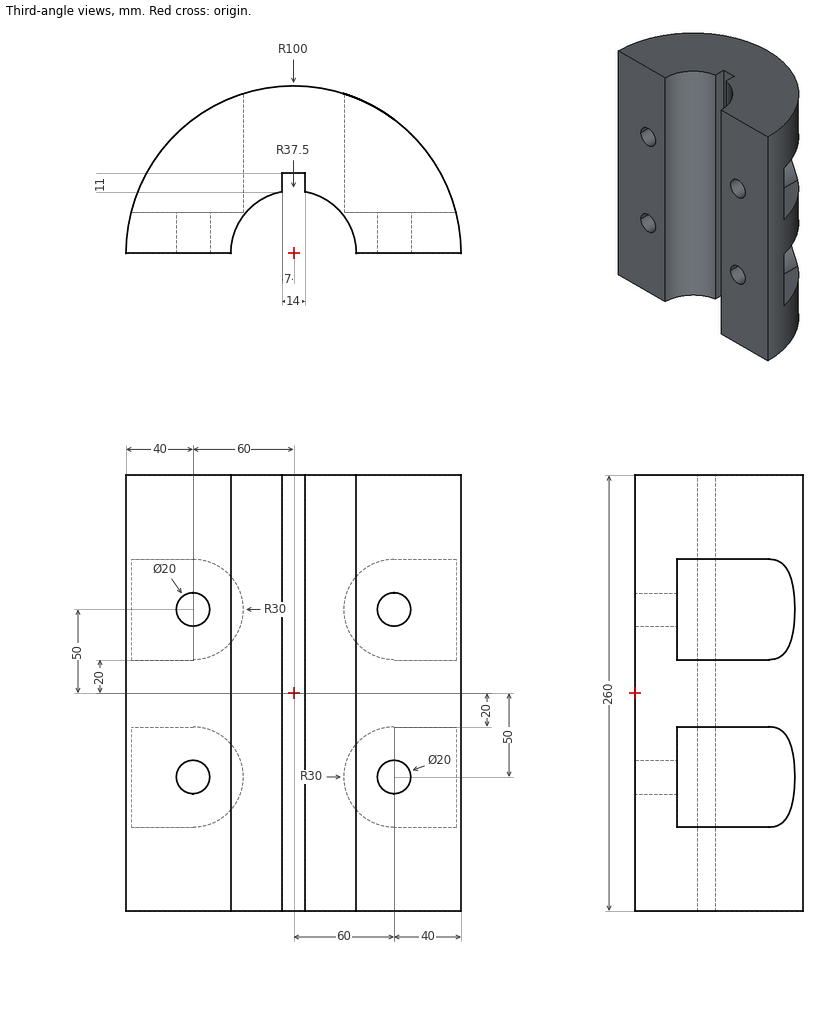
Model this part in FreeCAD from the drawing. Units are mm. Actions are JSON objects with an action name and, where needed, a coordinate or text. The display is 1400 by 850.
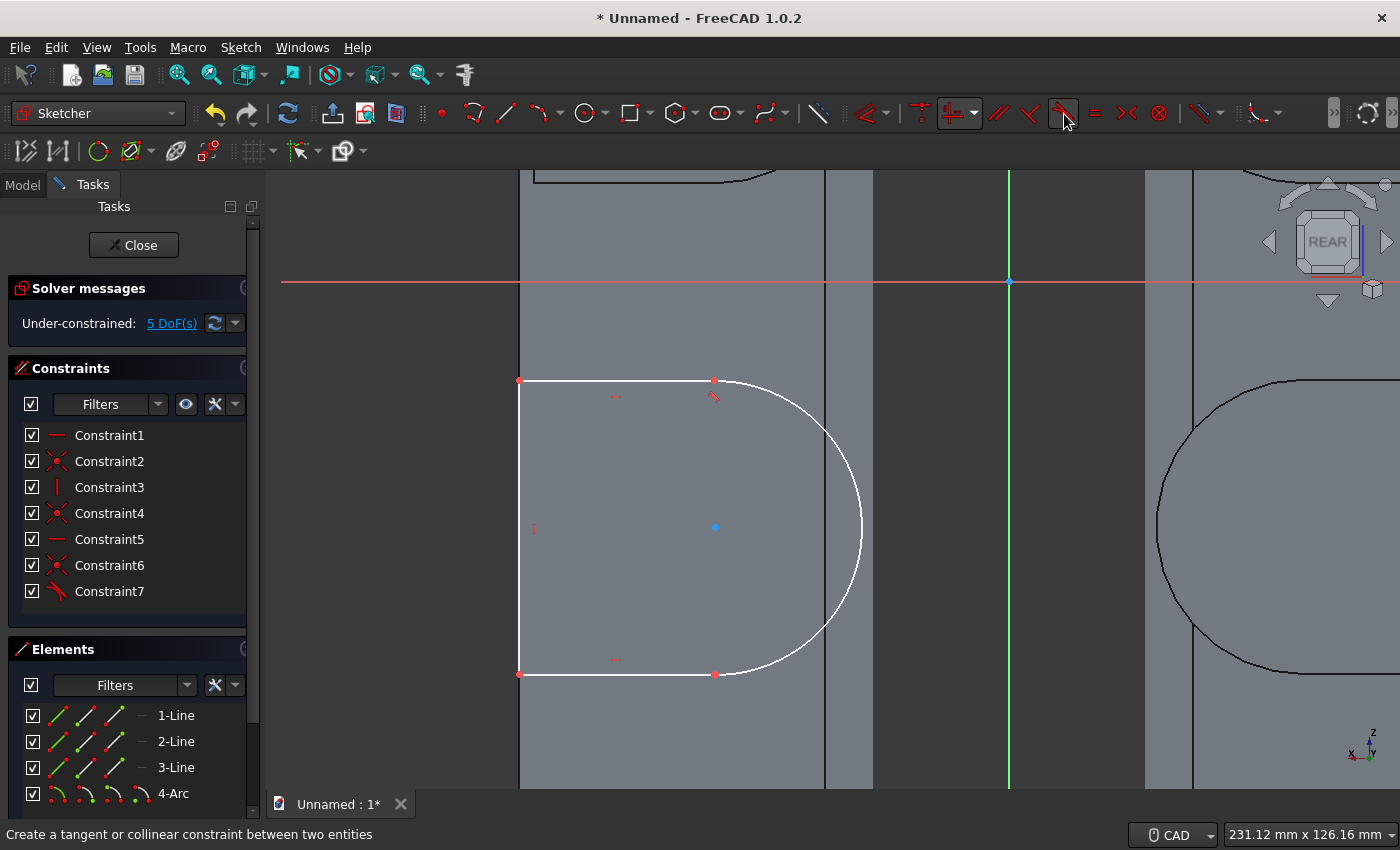
{"action": "left_click", "coordinate": [578, 675]}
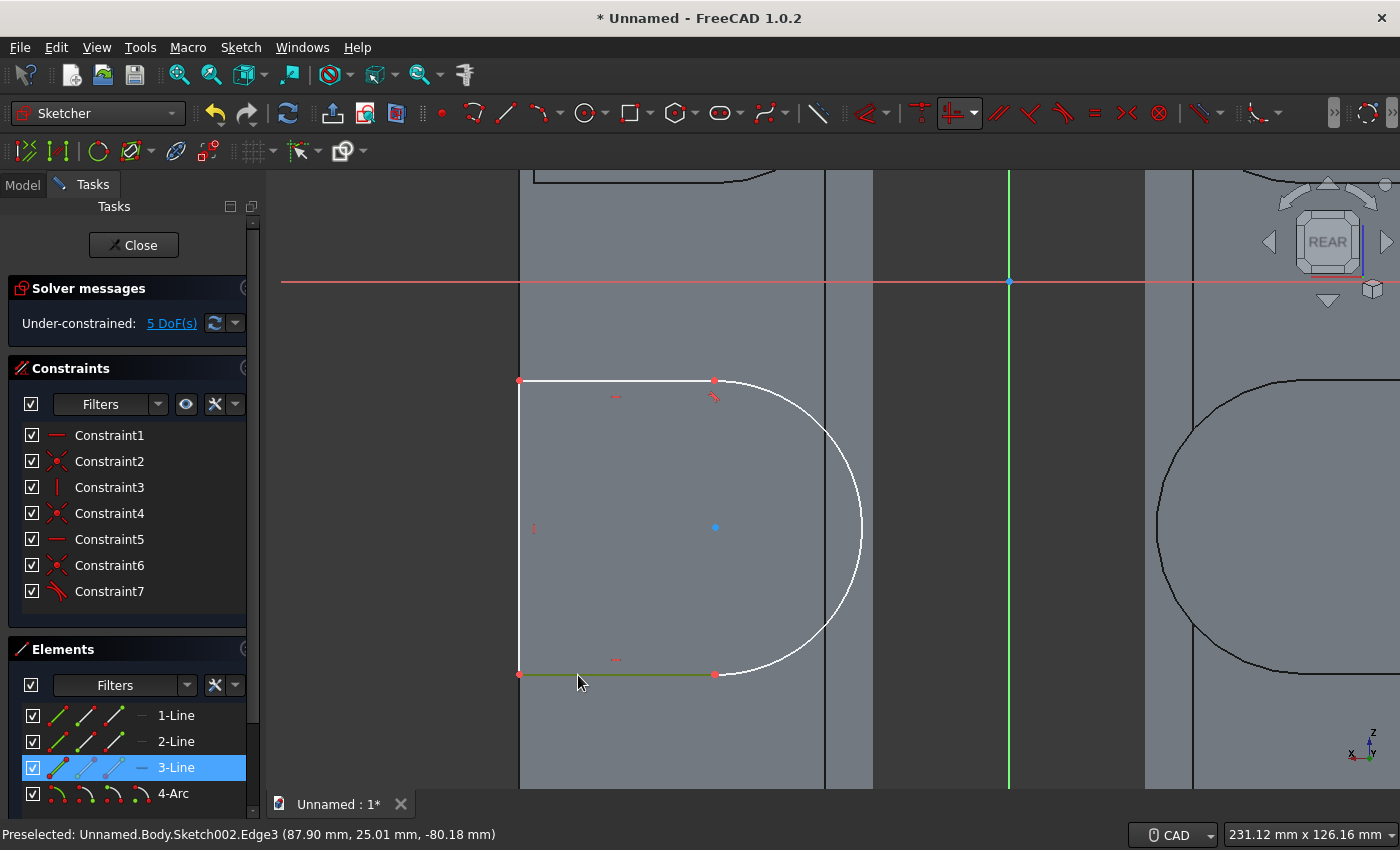
{"action": "left_click", "coordinate": [834, 614]}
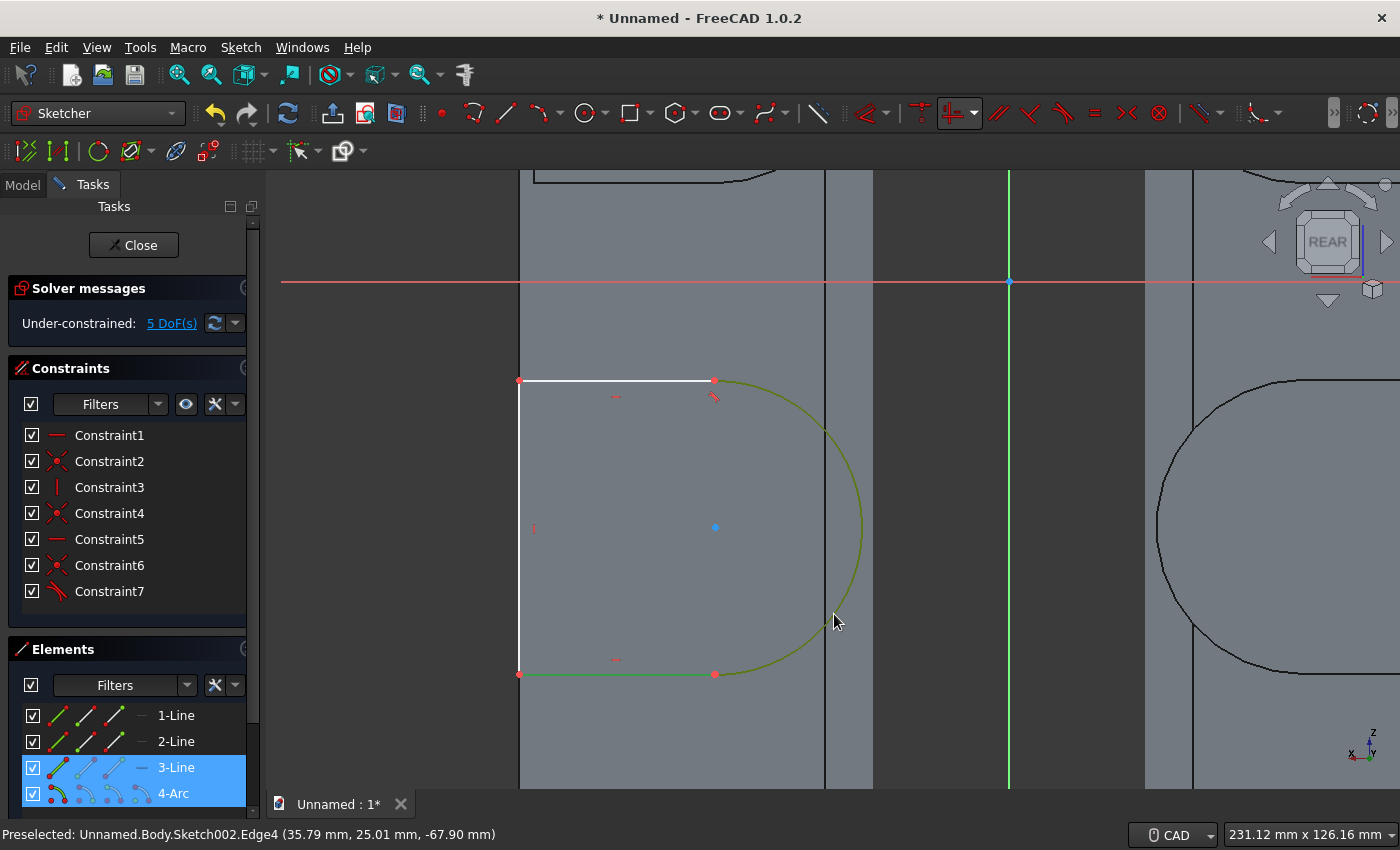
{"action": "left_click", "coordinate": [1064, 114]}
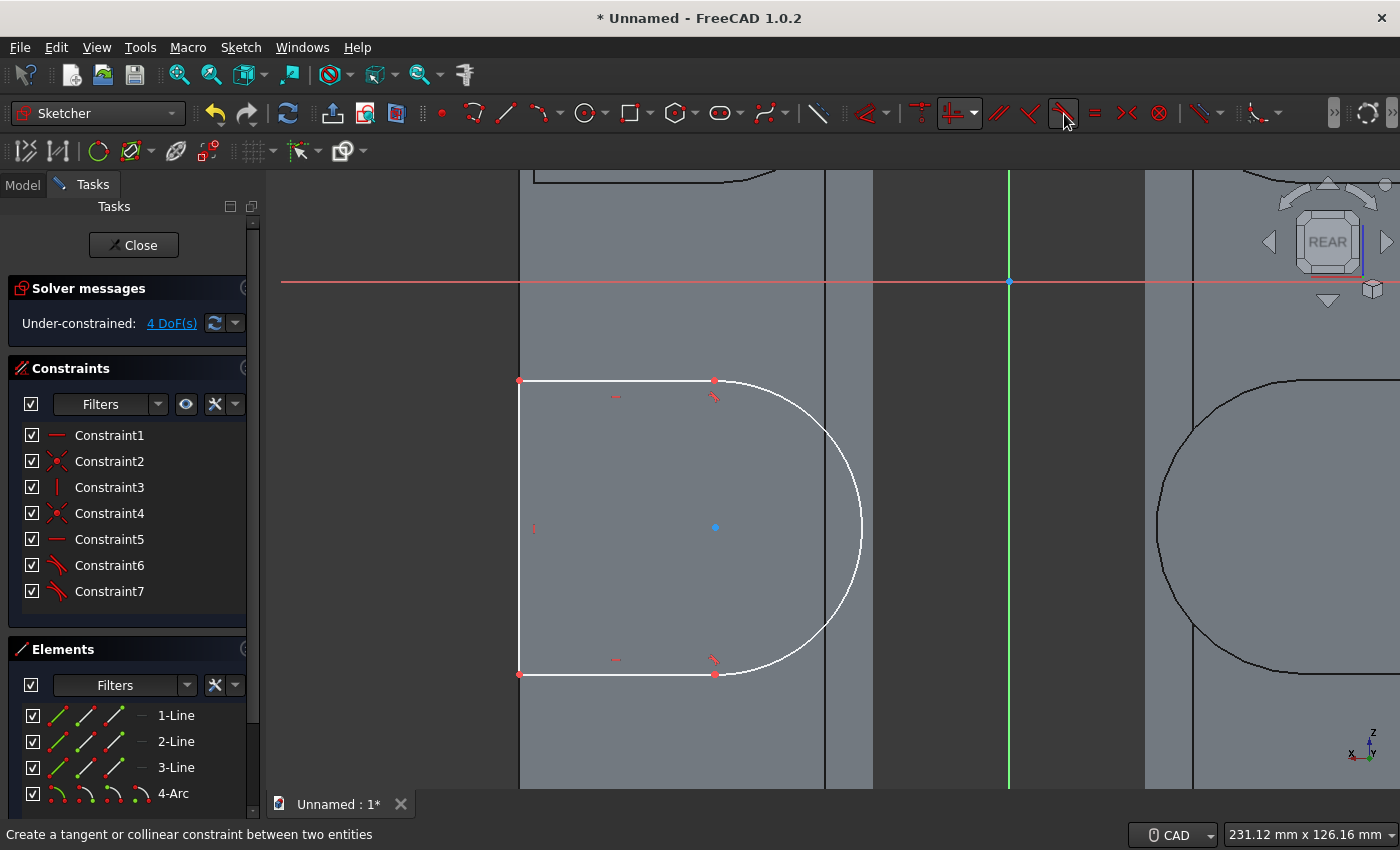
{"action": "left_click", "coordinate": [866, 114]}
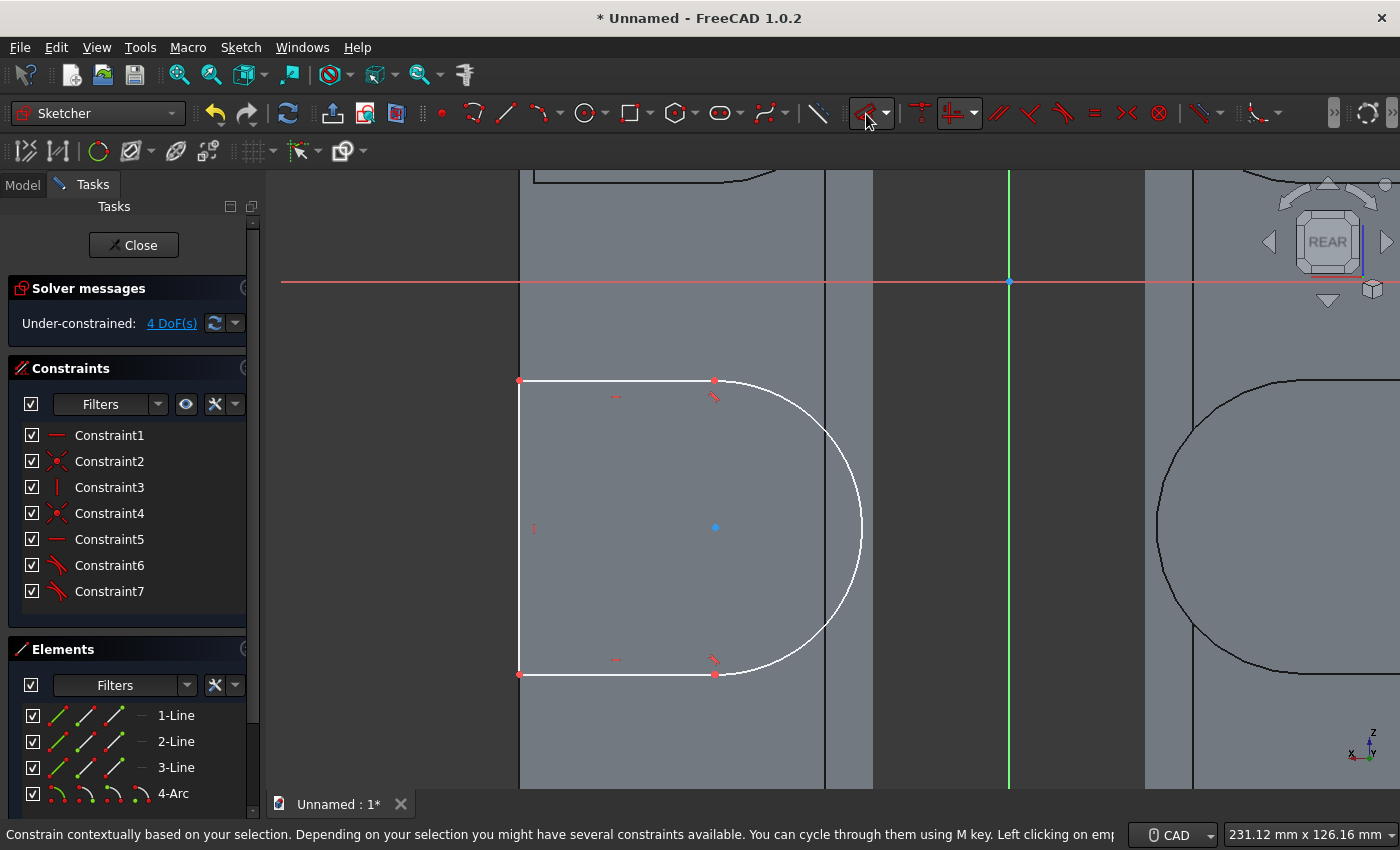
{"action": "left_click", "coordinate": [834, 614]}
{"action": "left_click", "coordinate": [860, 633]}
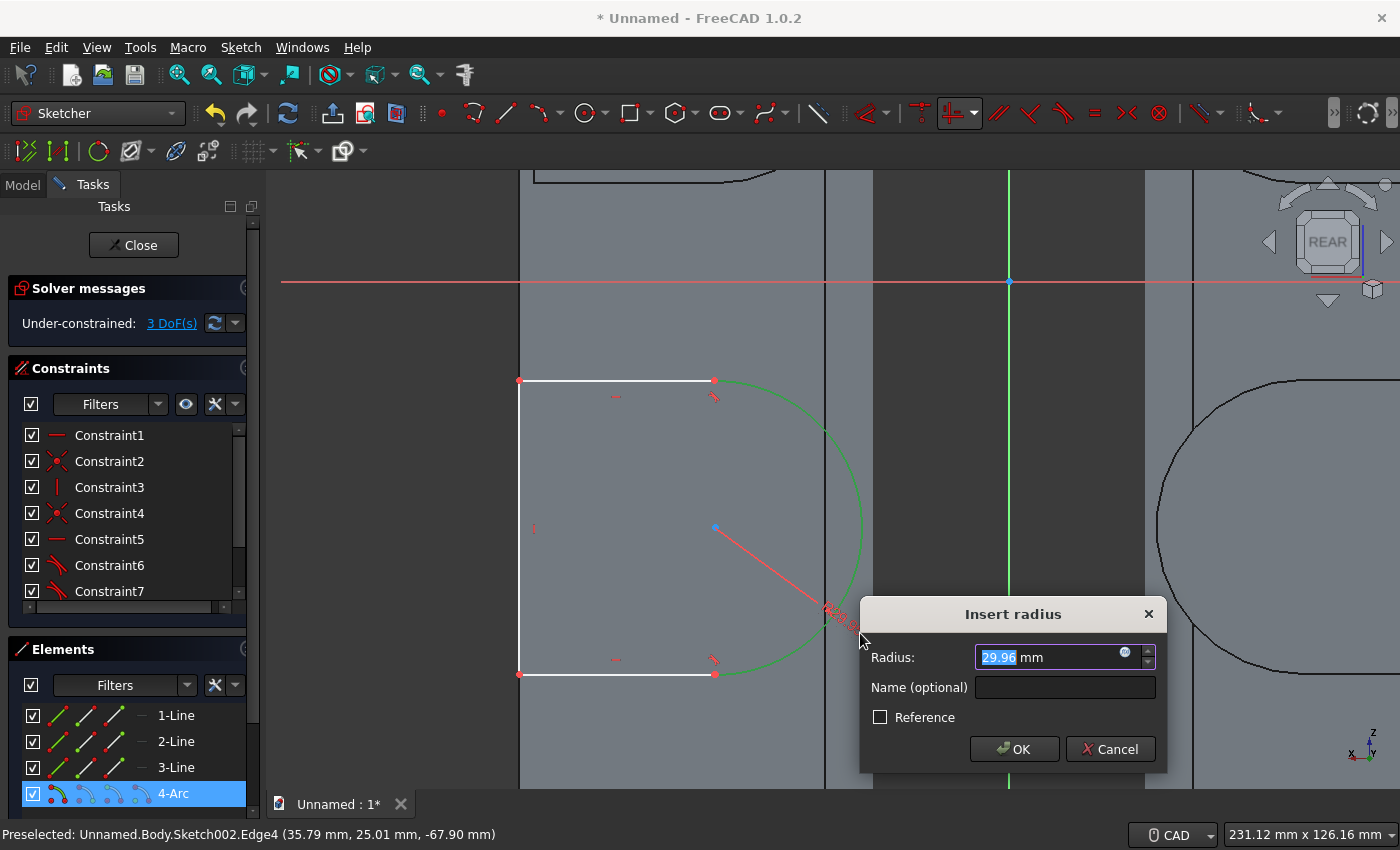
{"action": "type", "text": "30"}
{"action": "key", "text": "Return"}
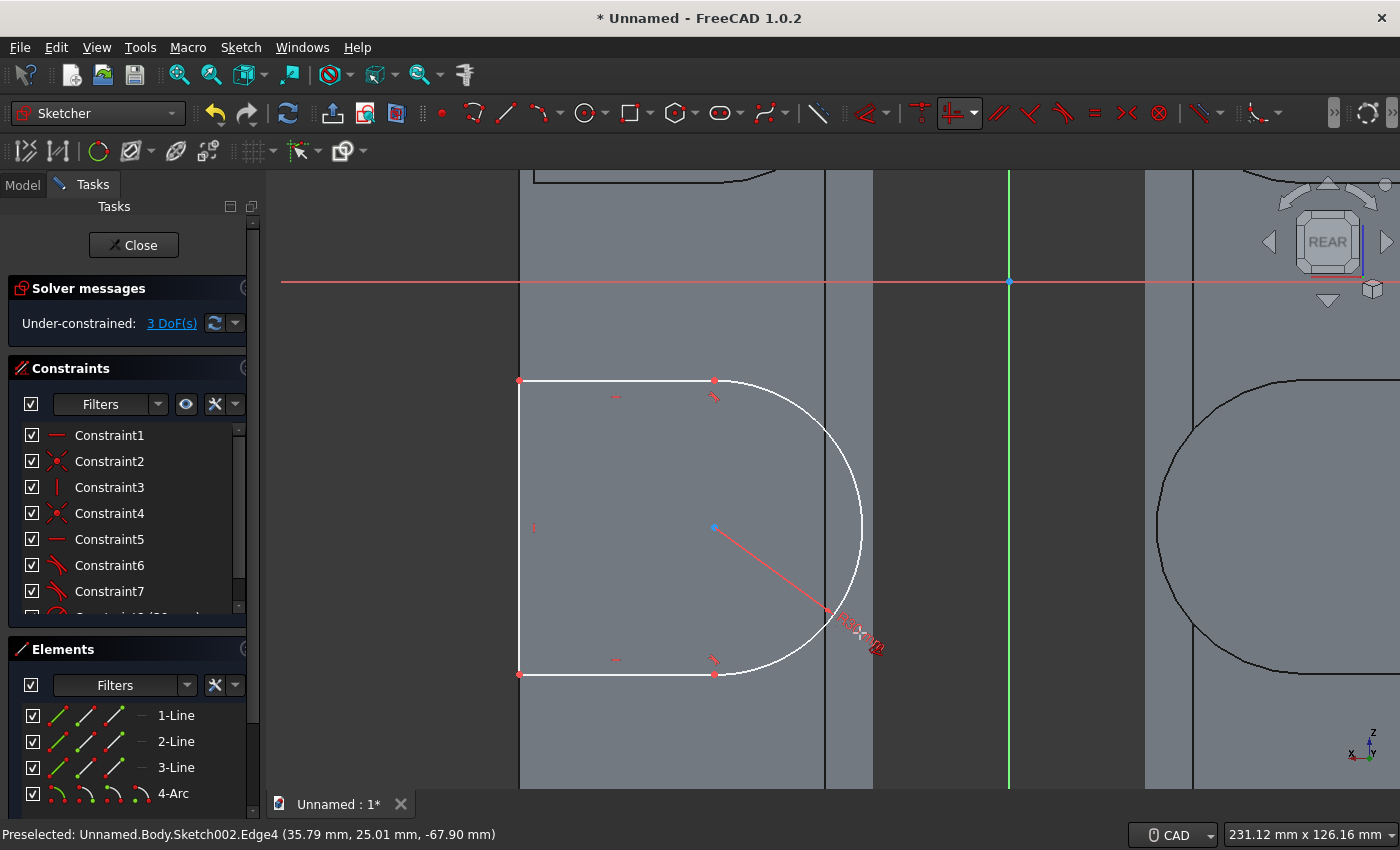
{"action": "left_click", "coordinate": [656, 381]}
{"action": "left_click", "coordinate": [617, 347]}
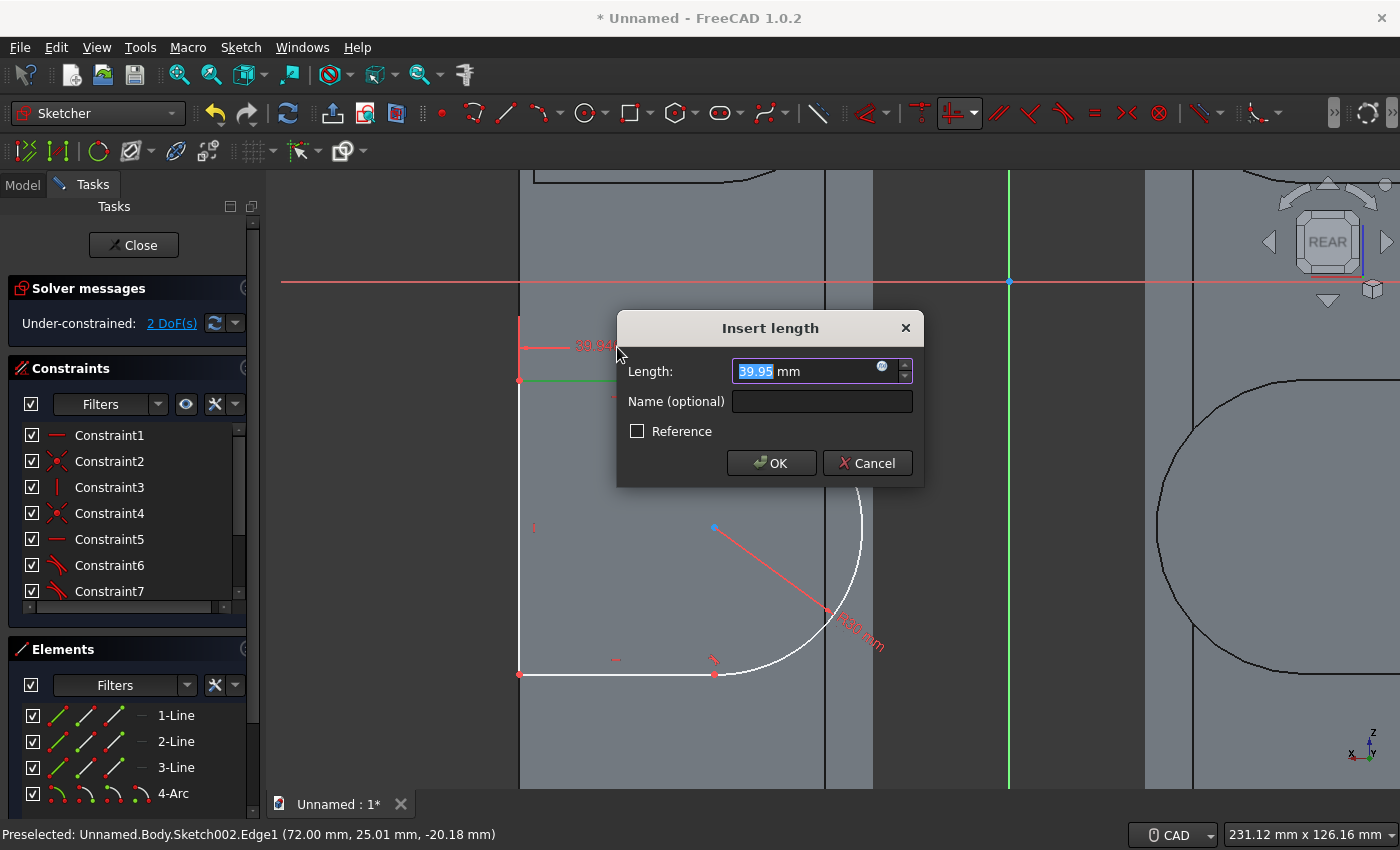
{"action": "type", "text": "40"}
{"action": "key", "text": "Return"}